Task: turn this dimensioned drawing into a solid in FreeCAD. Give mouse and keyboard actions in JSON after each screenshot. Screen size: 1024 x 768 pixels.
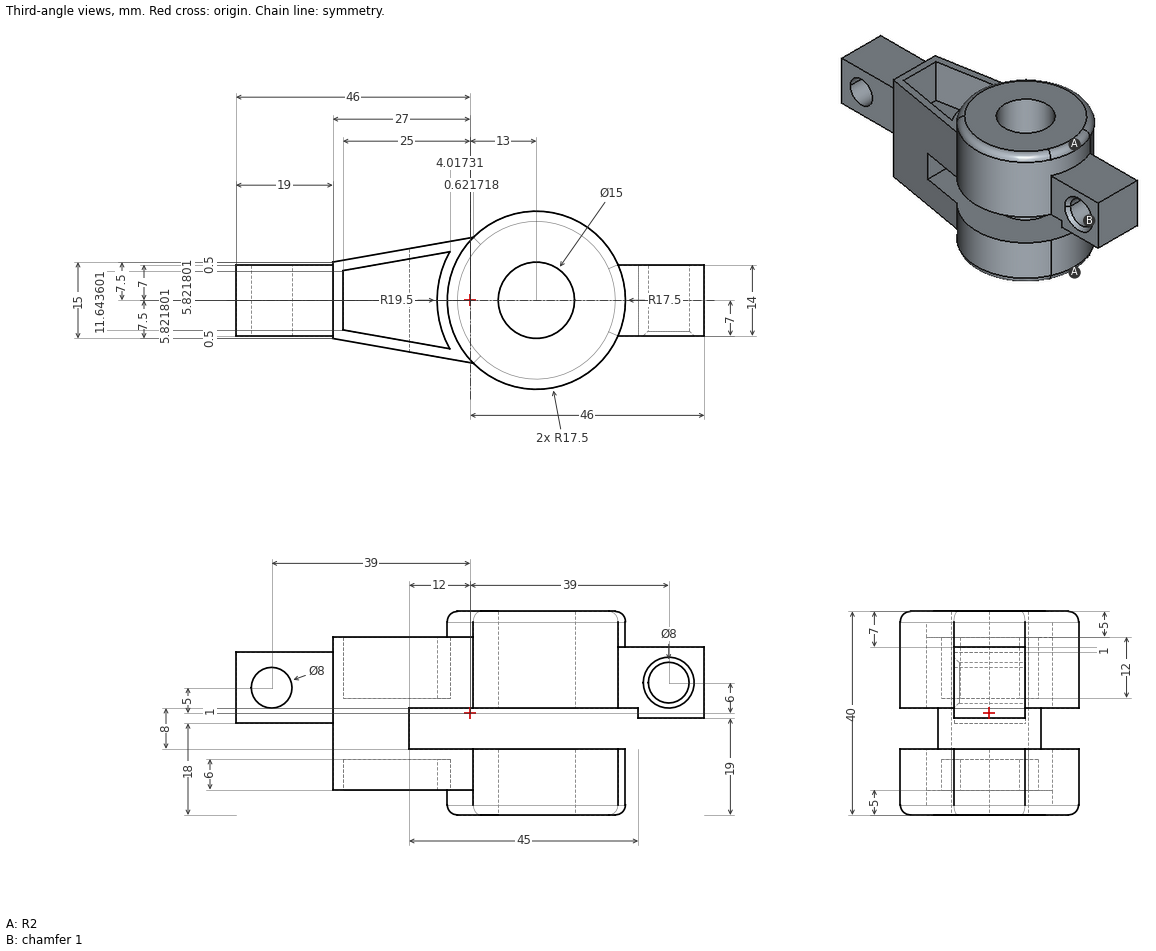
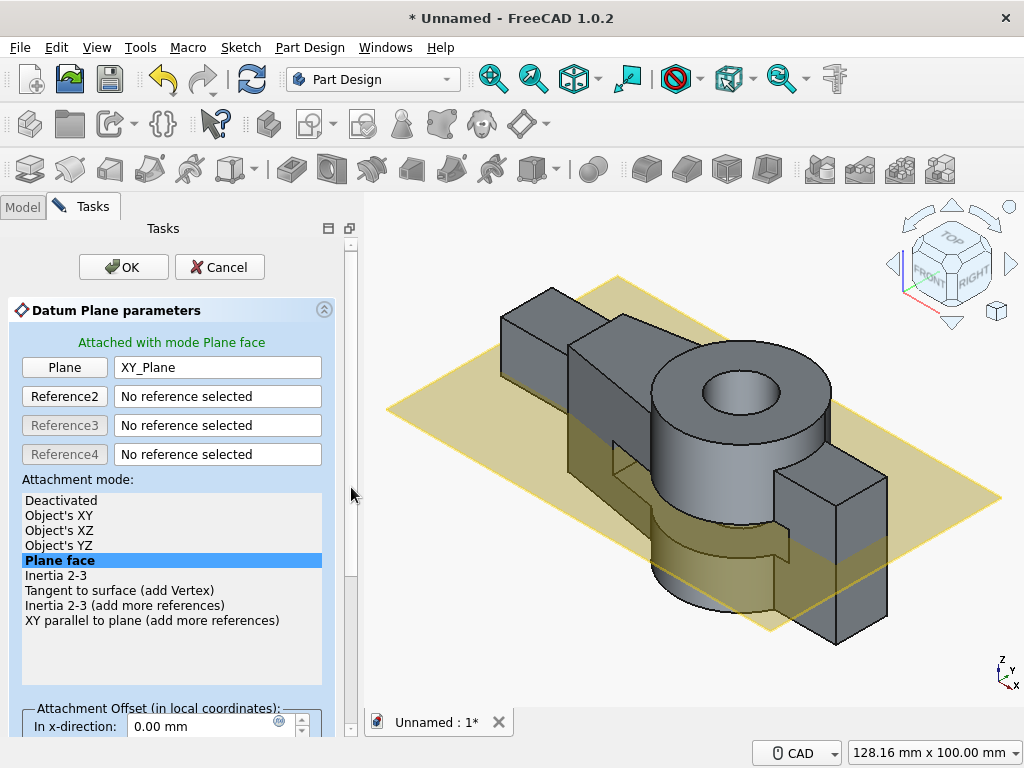
{"action": "left_click", "coordinate": [124, 267]}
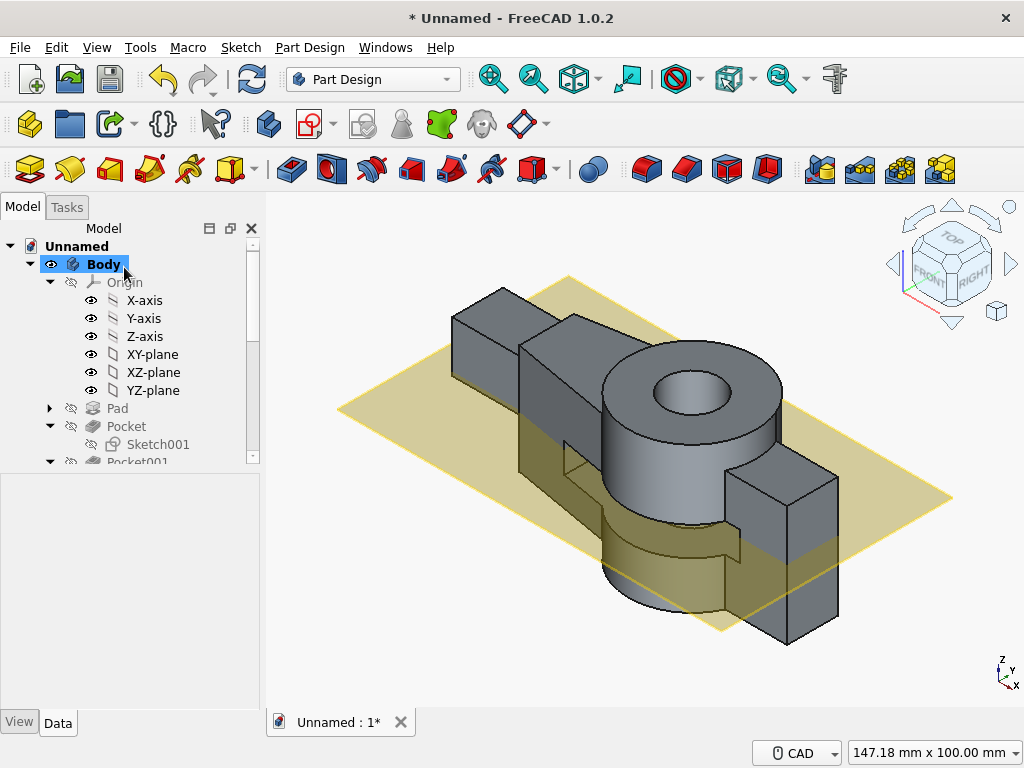
{"action": "scroll", "coordinate": [100, 350], "scroll_direction": "down", "scroll_amount": 3}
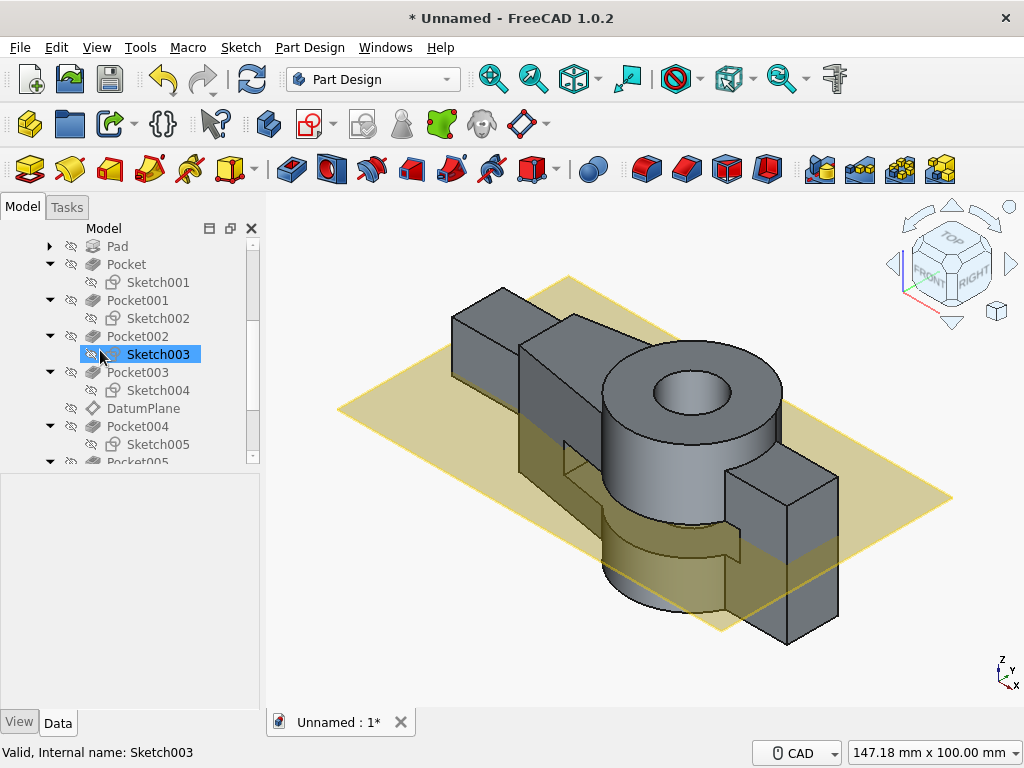
{"action": "scroll", "coordinate": [140, 350], "scroll_direction": "up", "scroll_amount": 15}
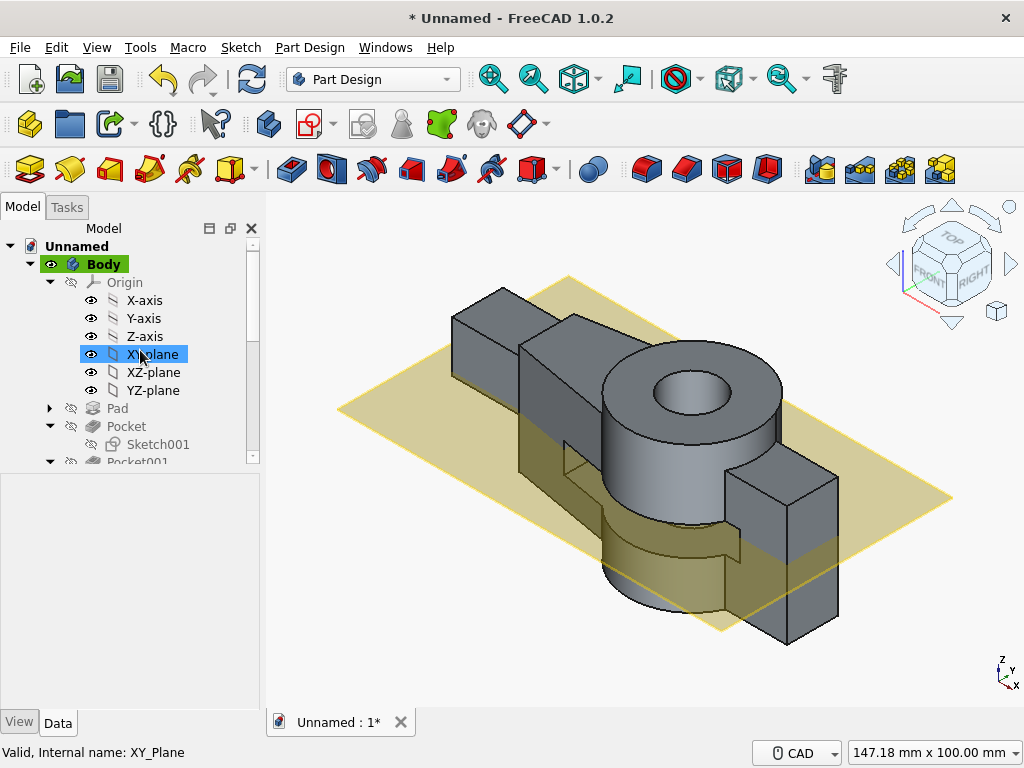
{"action": "scroll", "coordinate": [100, 350], "scroll_direction": "down", "scroll_amount": 6}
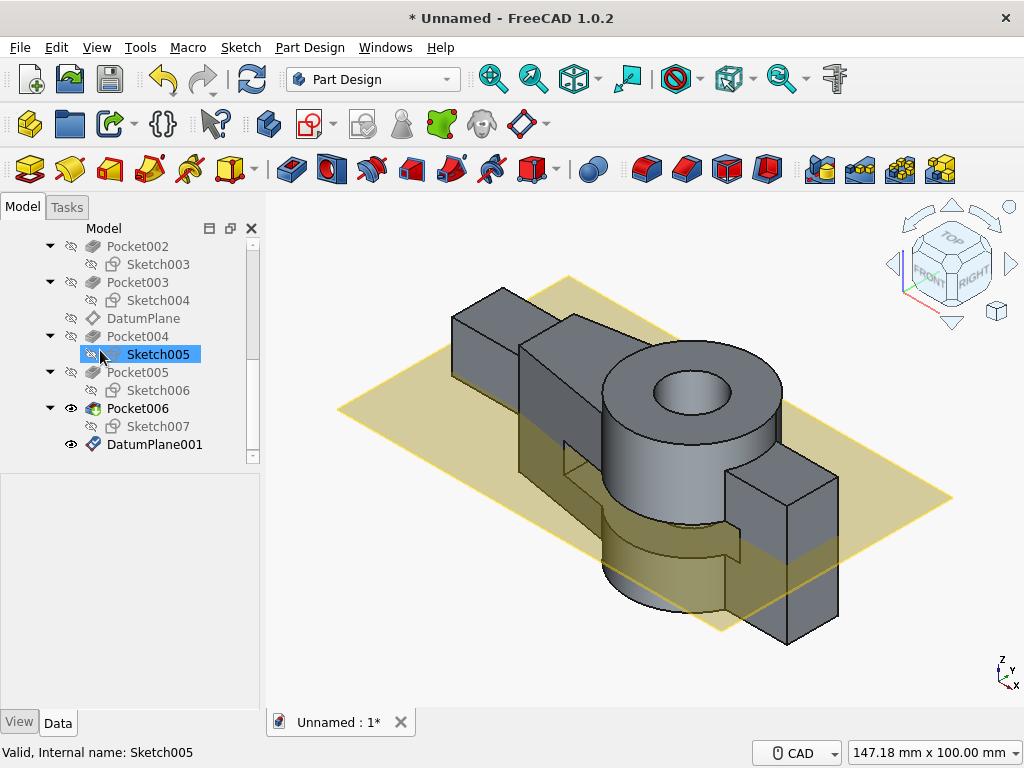
{"action": "left_click", "coordinate": [116, 444]}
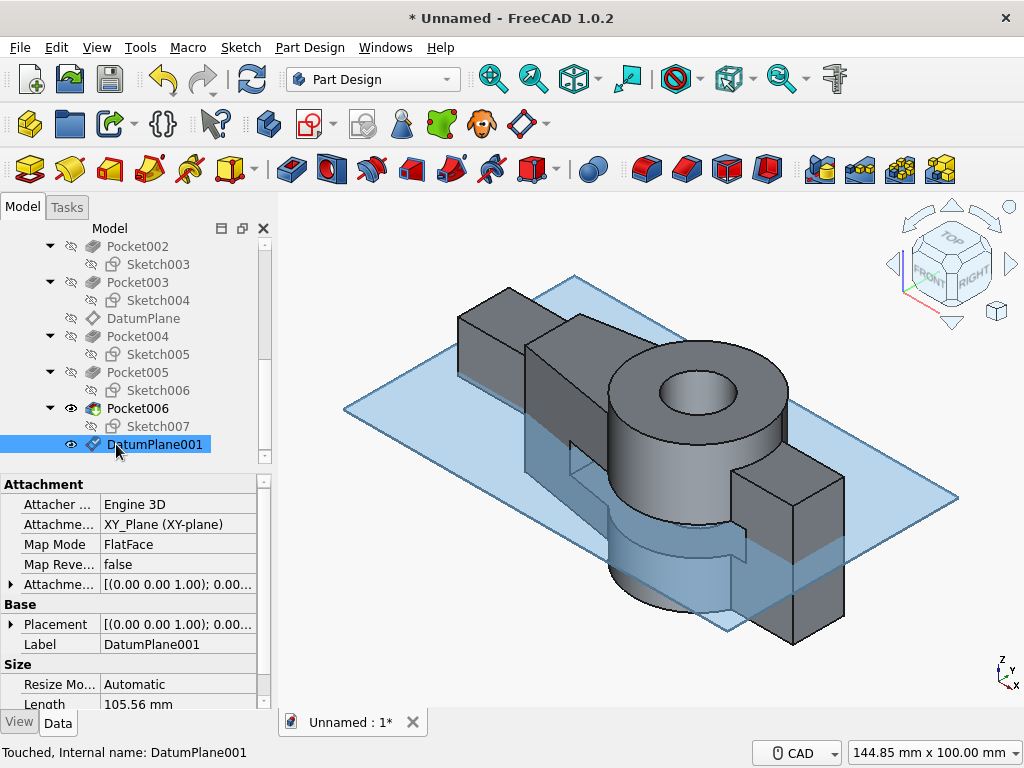
{"action": "left_click", "coordinate": [310, 124]}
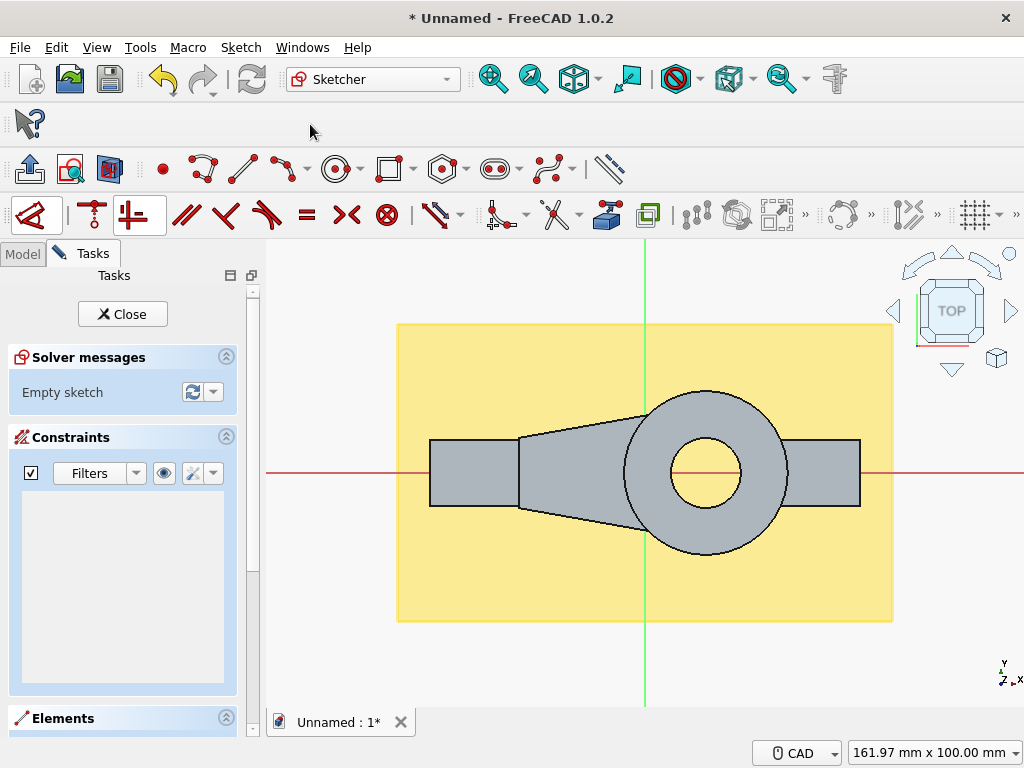
{"action": "left_click", "coordinate": [110, 170]}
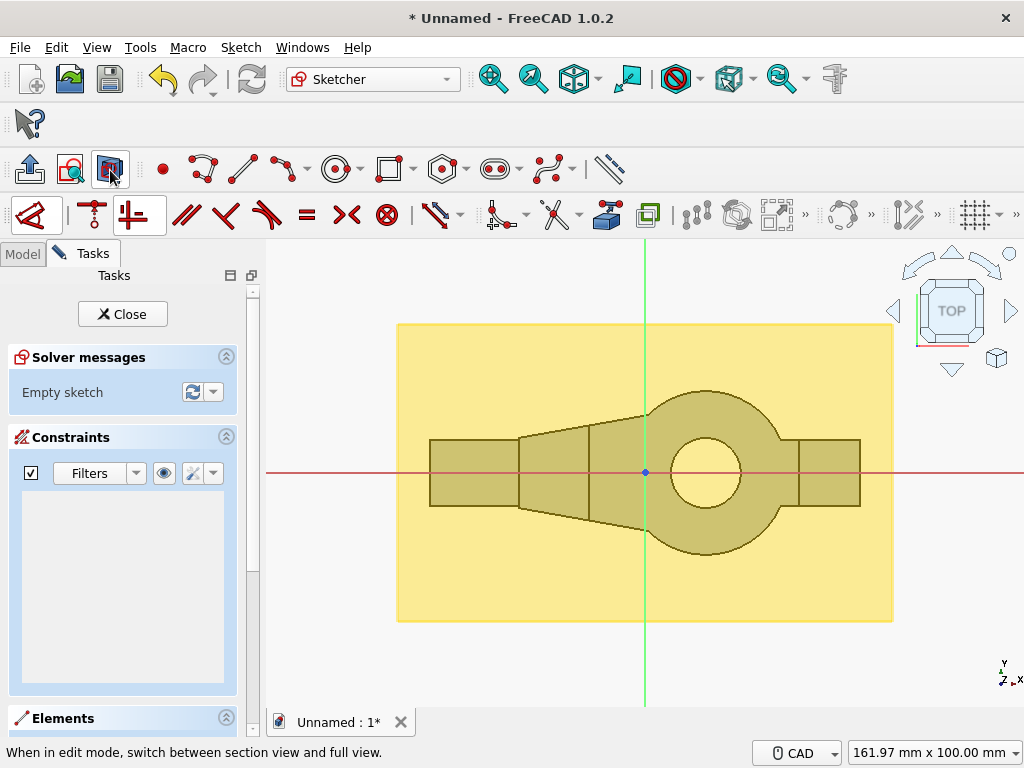
{"action": "scroll", "coordinate": [576, 473], "scroll_direction": "down", "scroll_amount": 5}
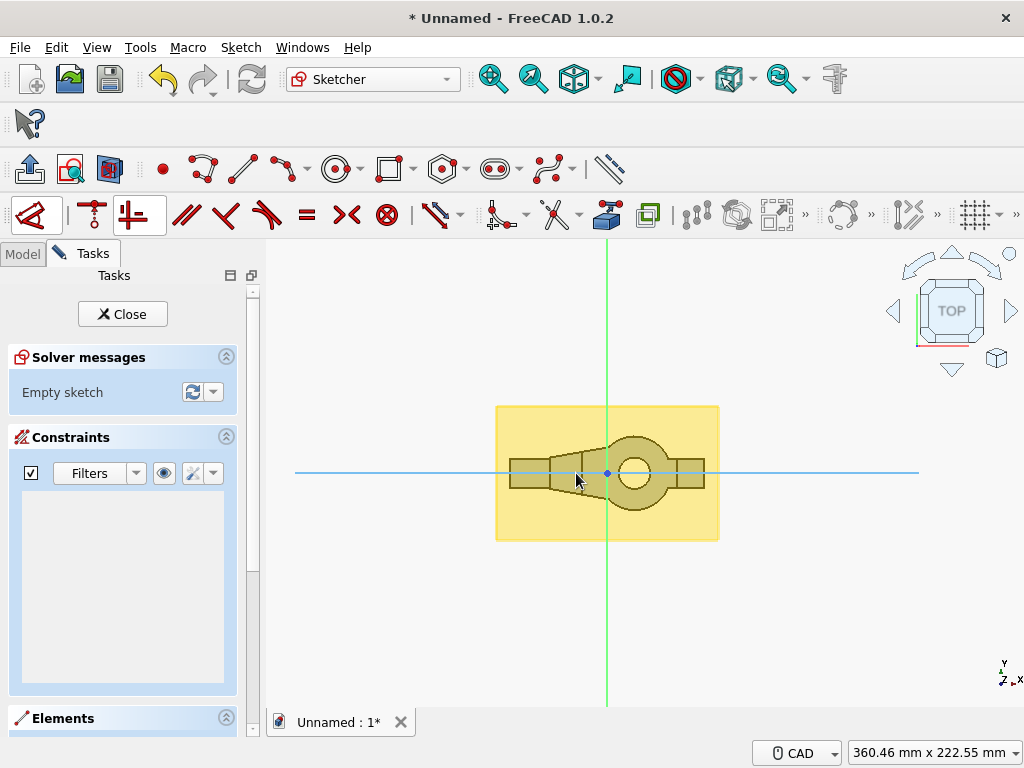
{"action": "scroll", "coordinate": [675, 473], "scroll_direction": "up", "scroll_amount": 12}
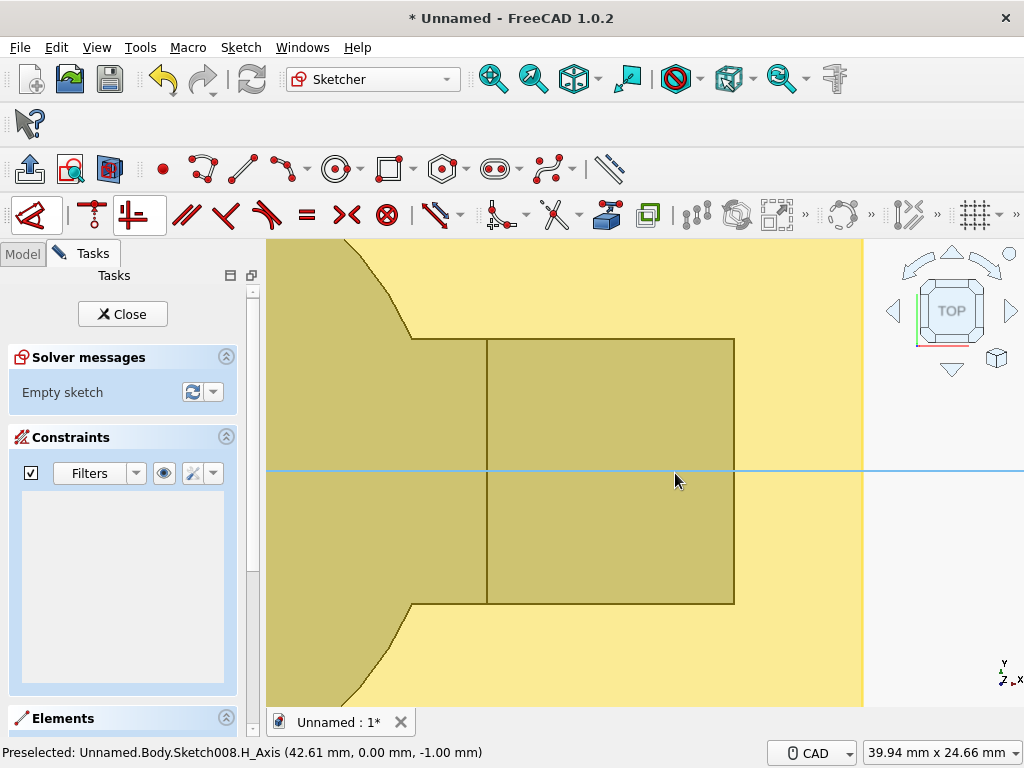
{"action": "left_click", "coordinate": [204, 170]}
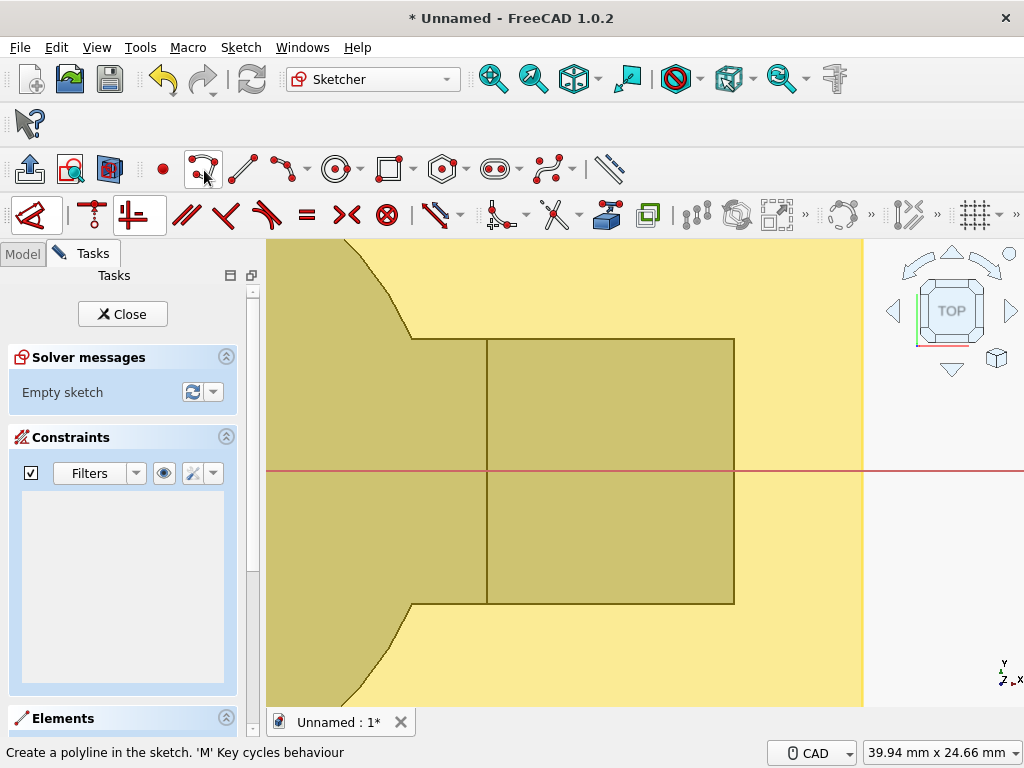
{"action": "left_click", "coordinate": [412, 339]}
{"action": "left_click", "coordinate": [734, 339]}
{"action": "left_click", "coordinate": [734, 604]}
{"action": "left_click", "coordinate": [412, 604]}
{"action": "right_click", "coordinate": [412, 604]}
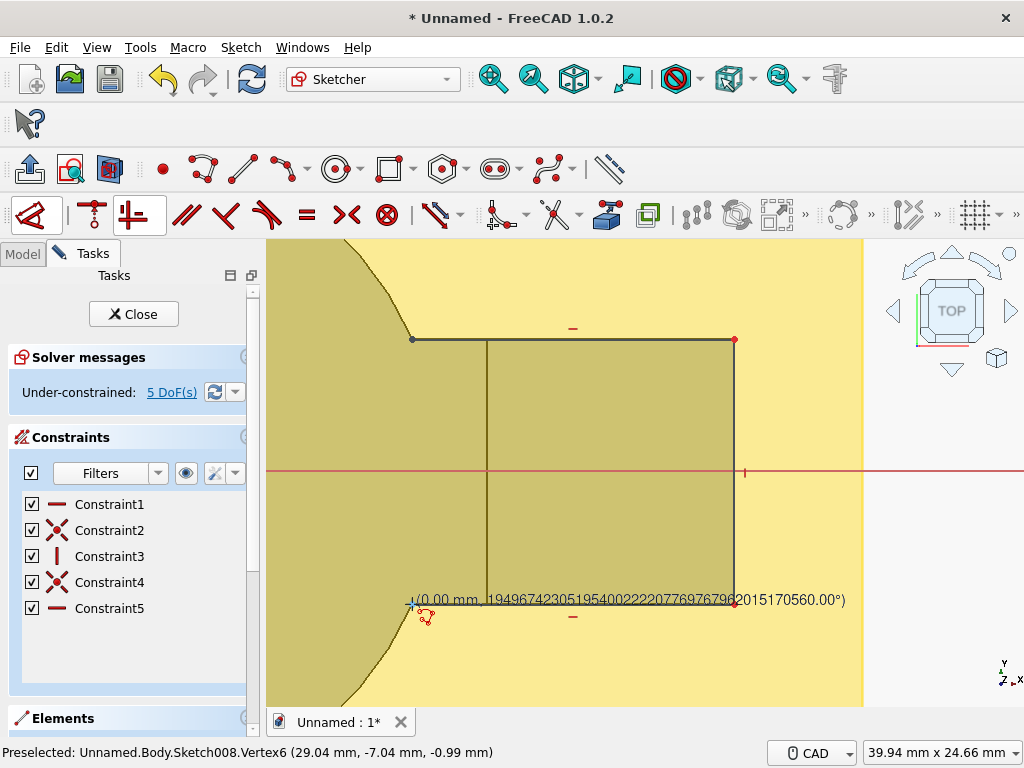
{"action": "left_click", "coordinate": [284, 170]}